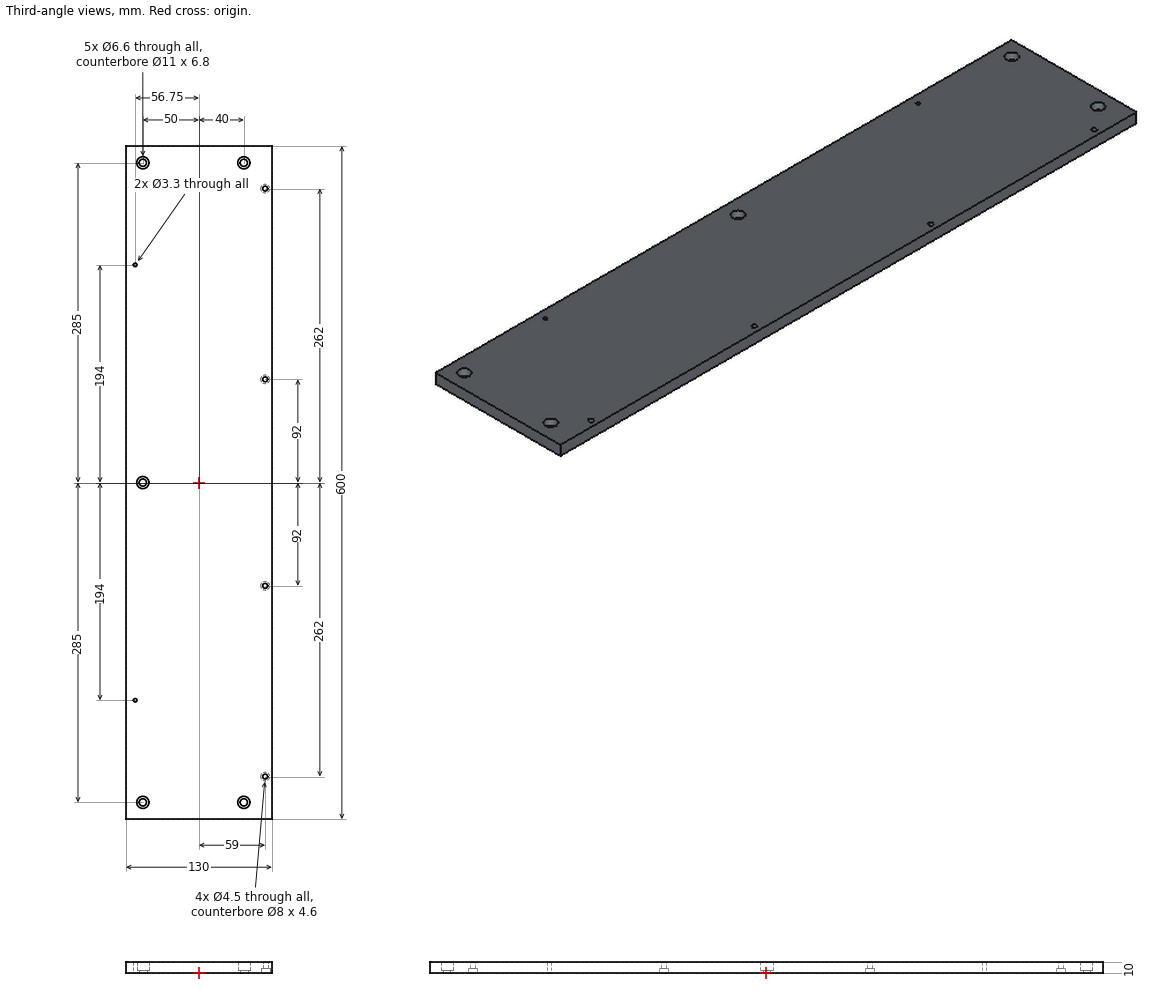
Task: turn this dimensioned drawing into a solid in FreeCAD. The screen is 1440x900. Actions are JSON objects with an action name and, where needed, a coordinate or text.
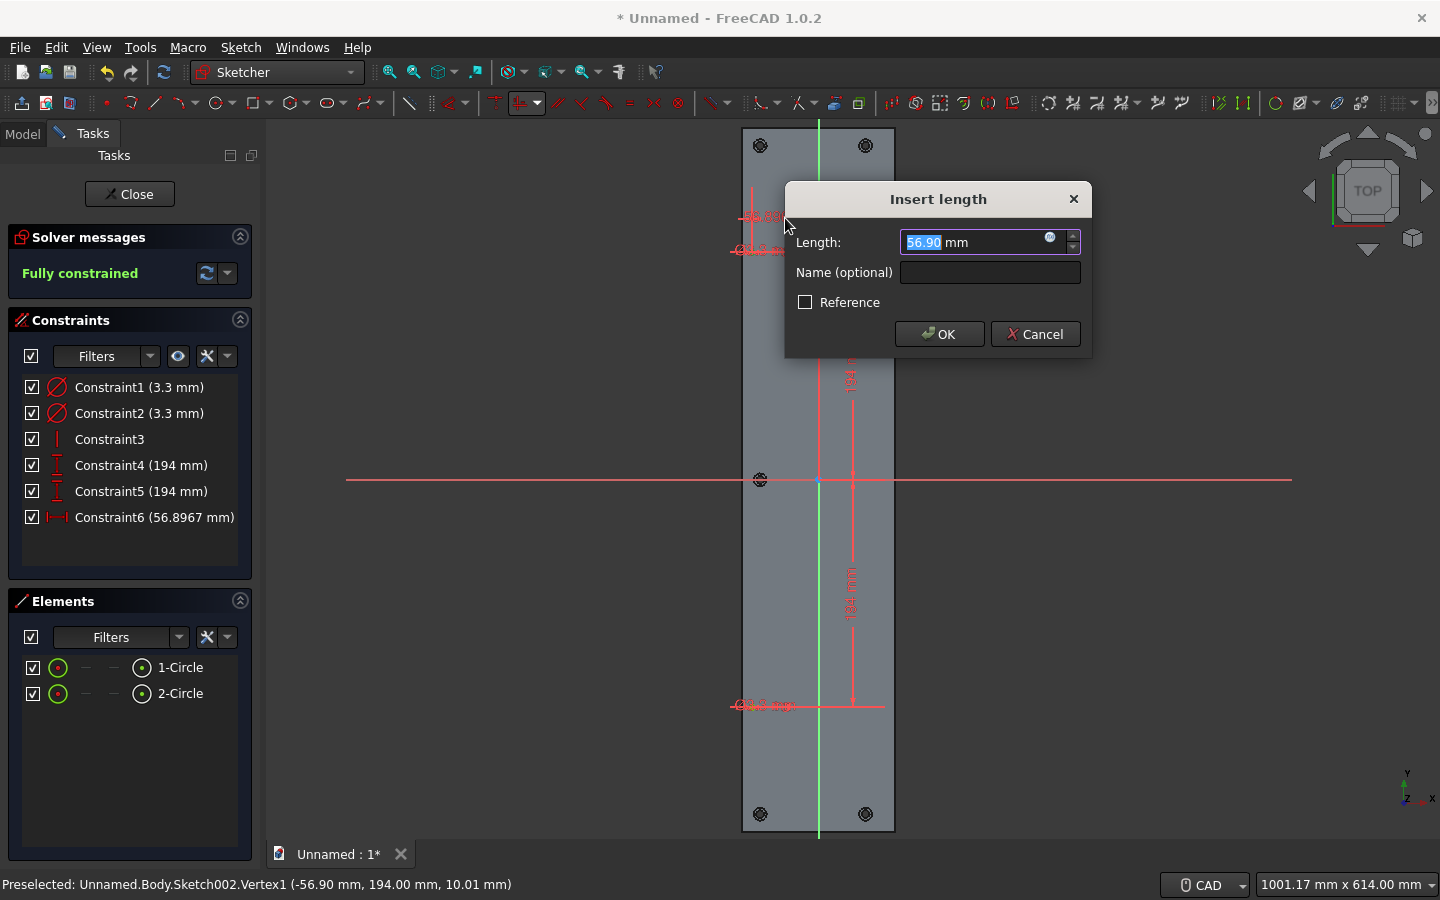
{"action": "type", "text": "56.75"}
{"action": "key", "text": "Return"}
{"action": "key", "text": "Escape"}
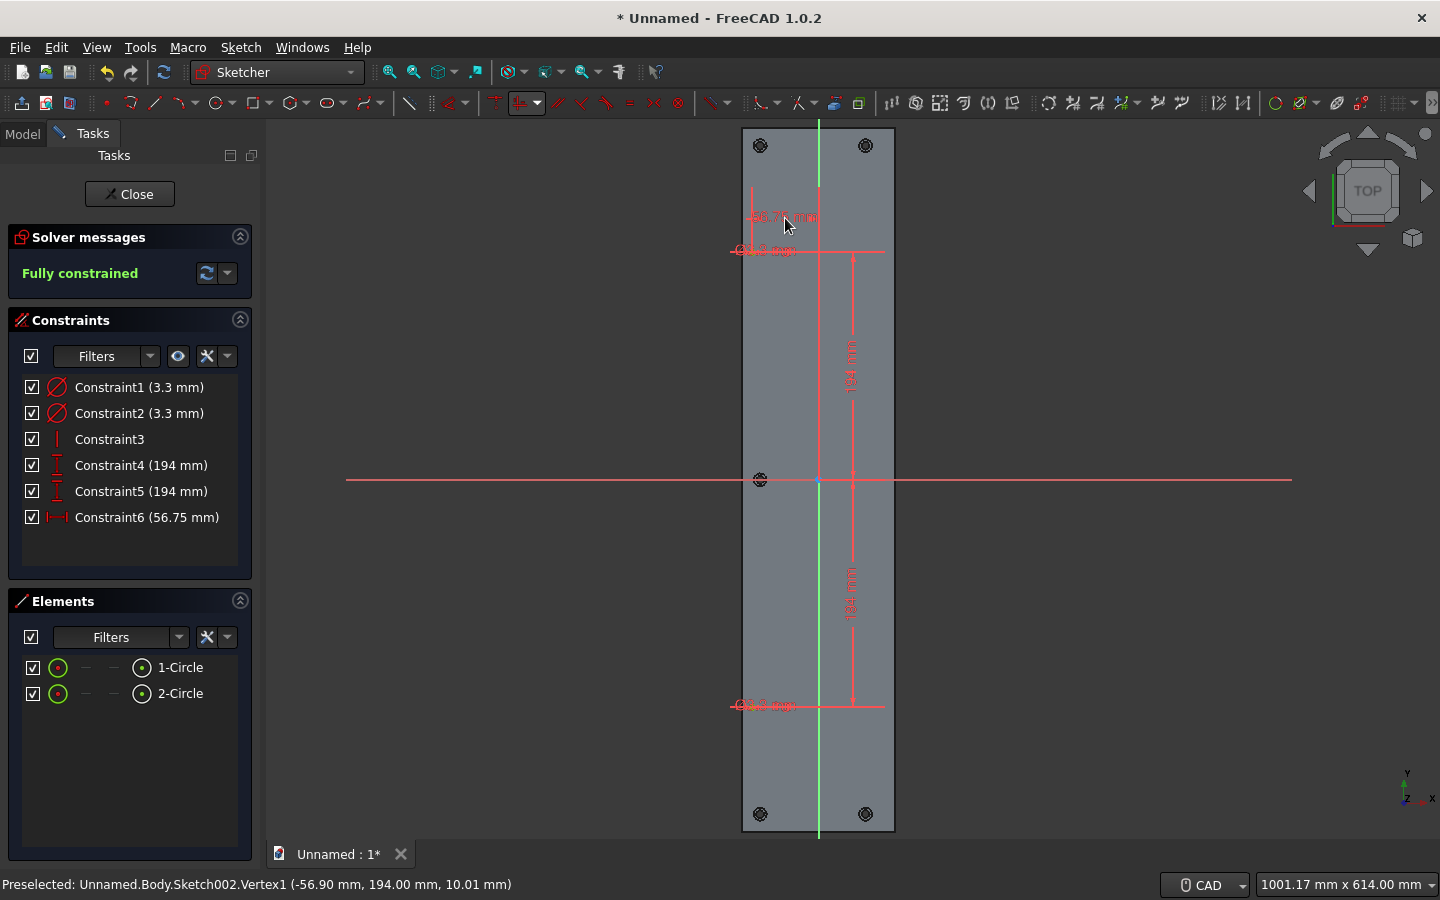
{"action": "left_click", "coordinate": [130, 194]}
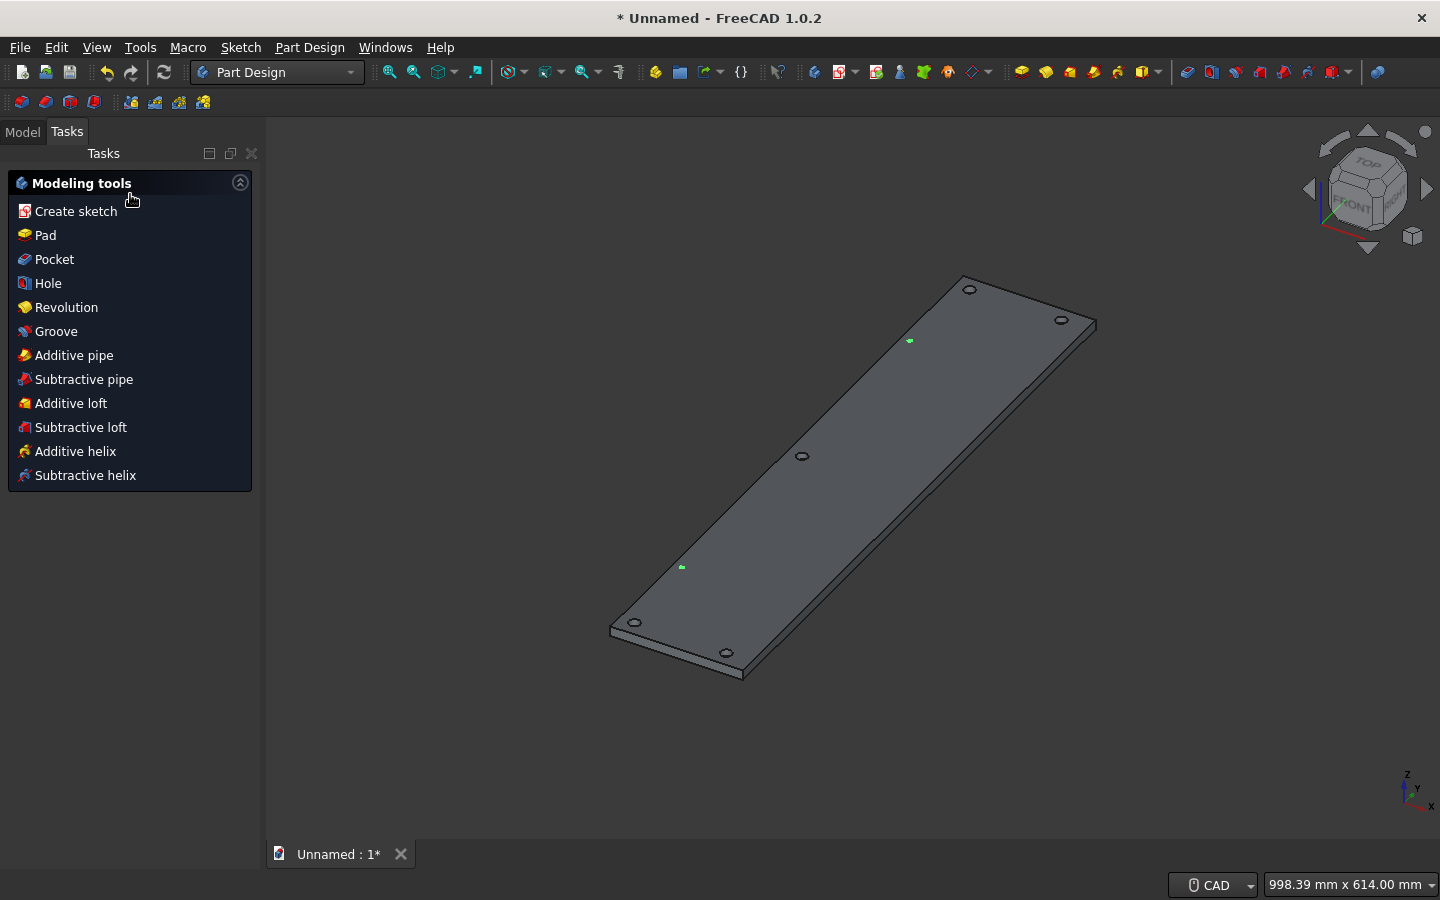
{"action": "left_click", "coordinate": [1212, 72]}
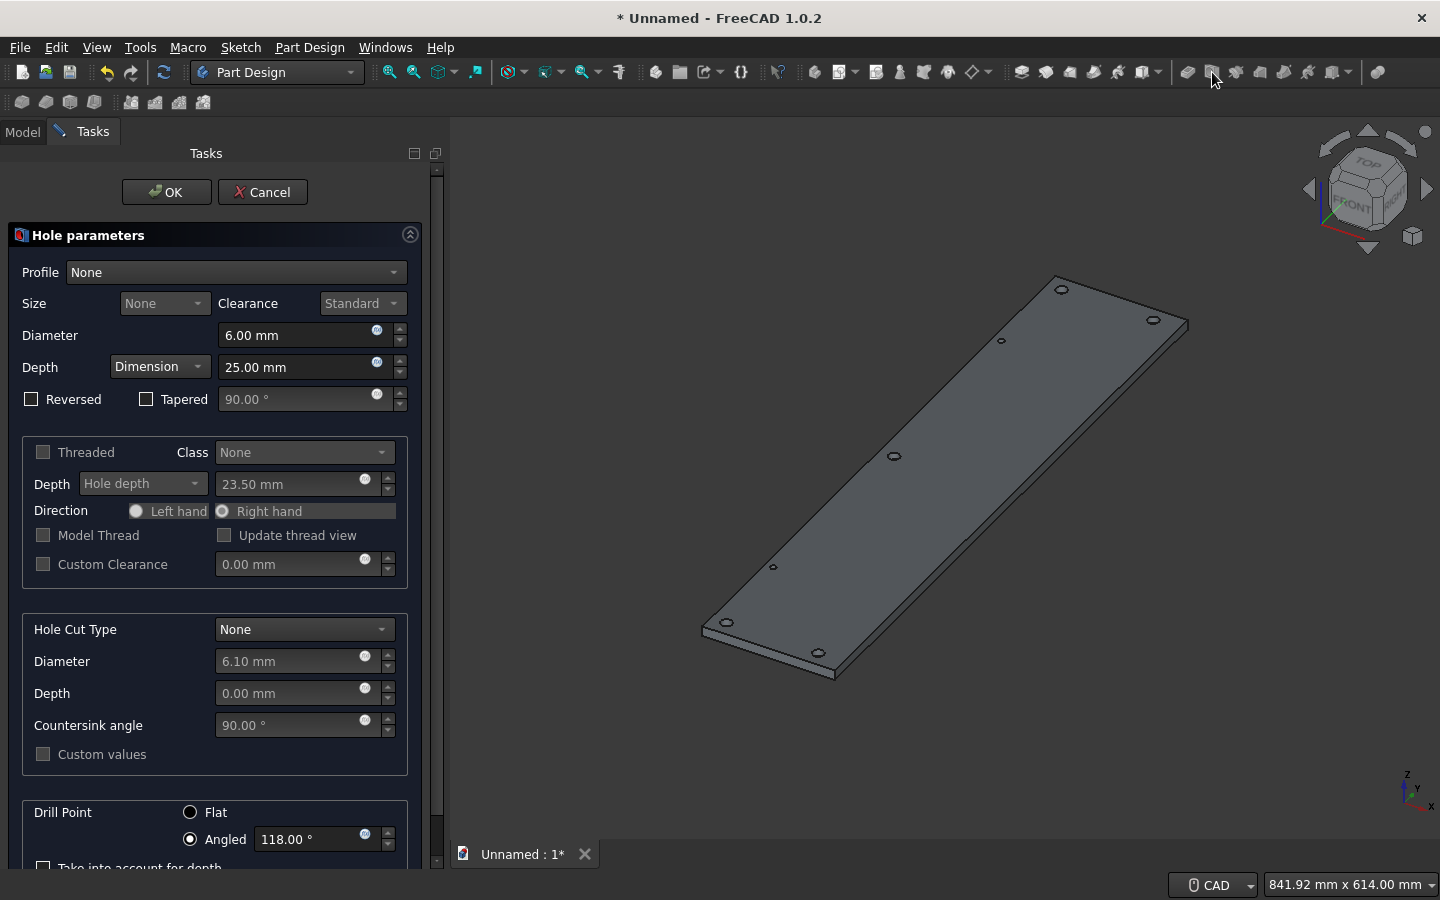
{"action": "triple_click", "coordinate": [305, 335]}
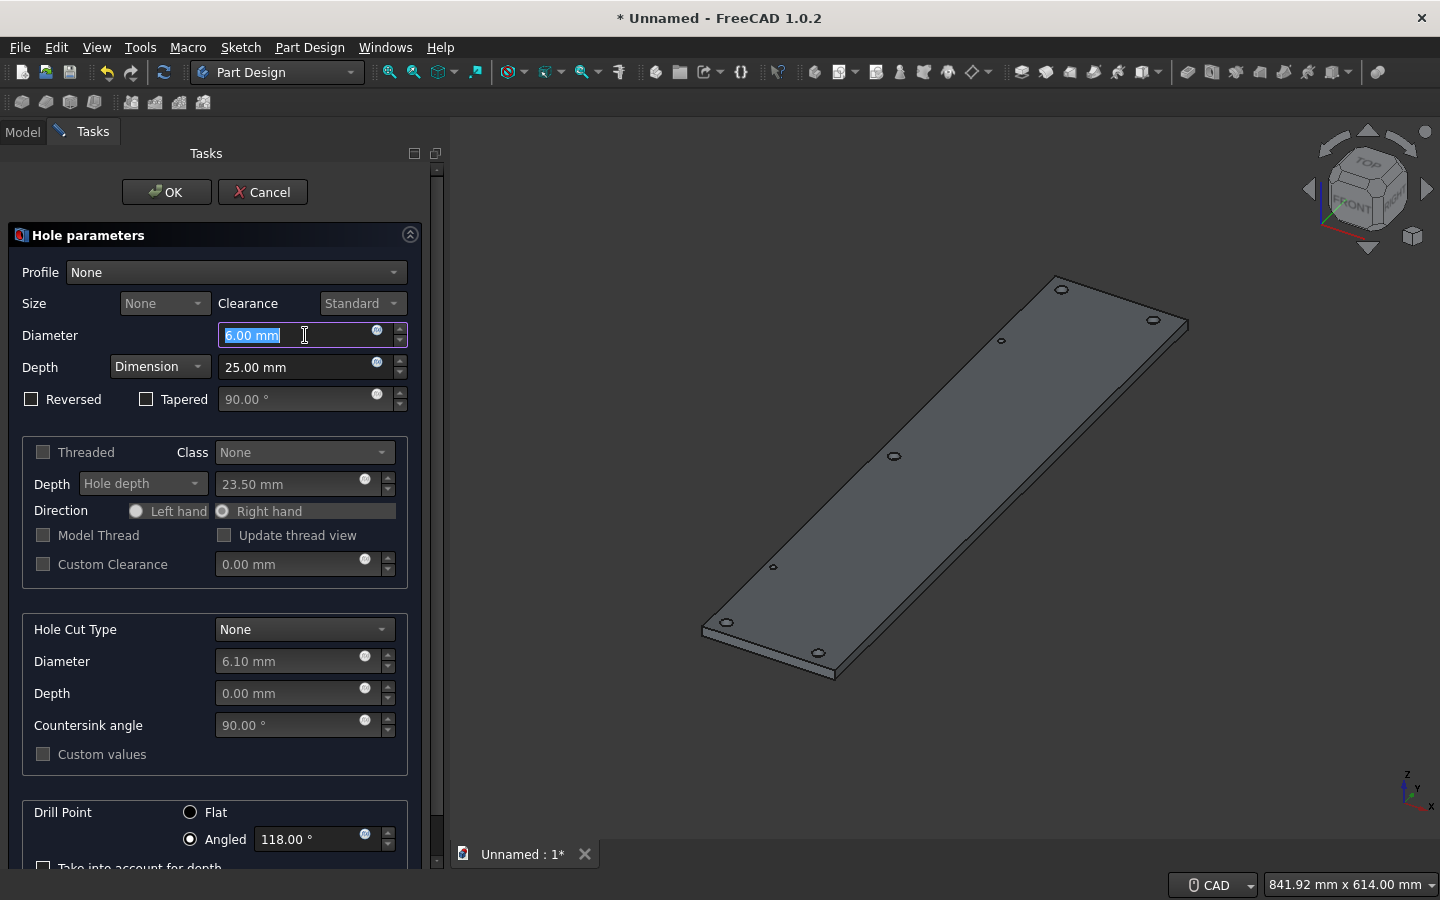
{"action": "type", "text": "3.3"}
{"action": "key", "text": "Tab"}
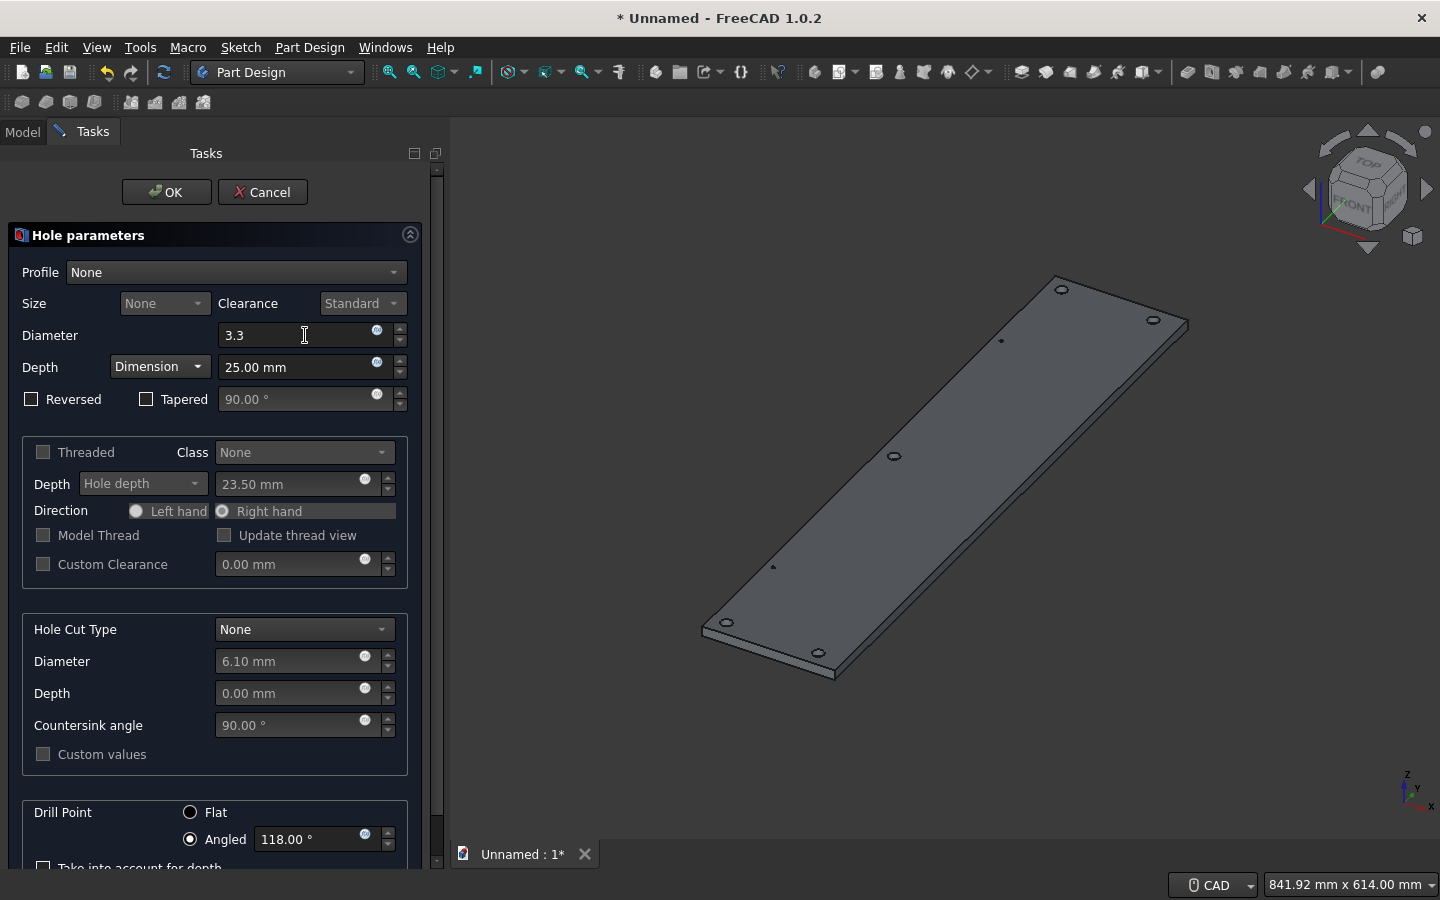
{"action": "left_click", "coordinate": [161, 366]}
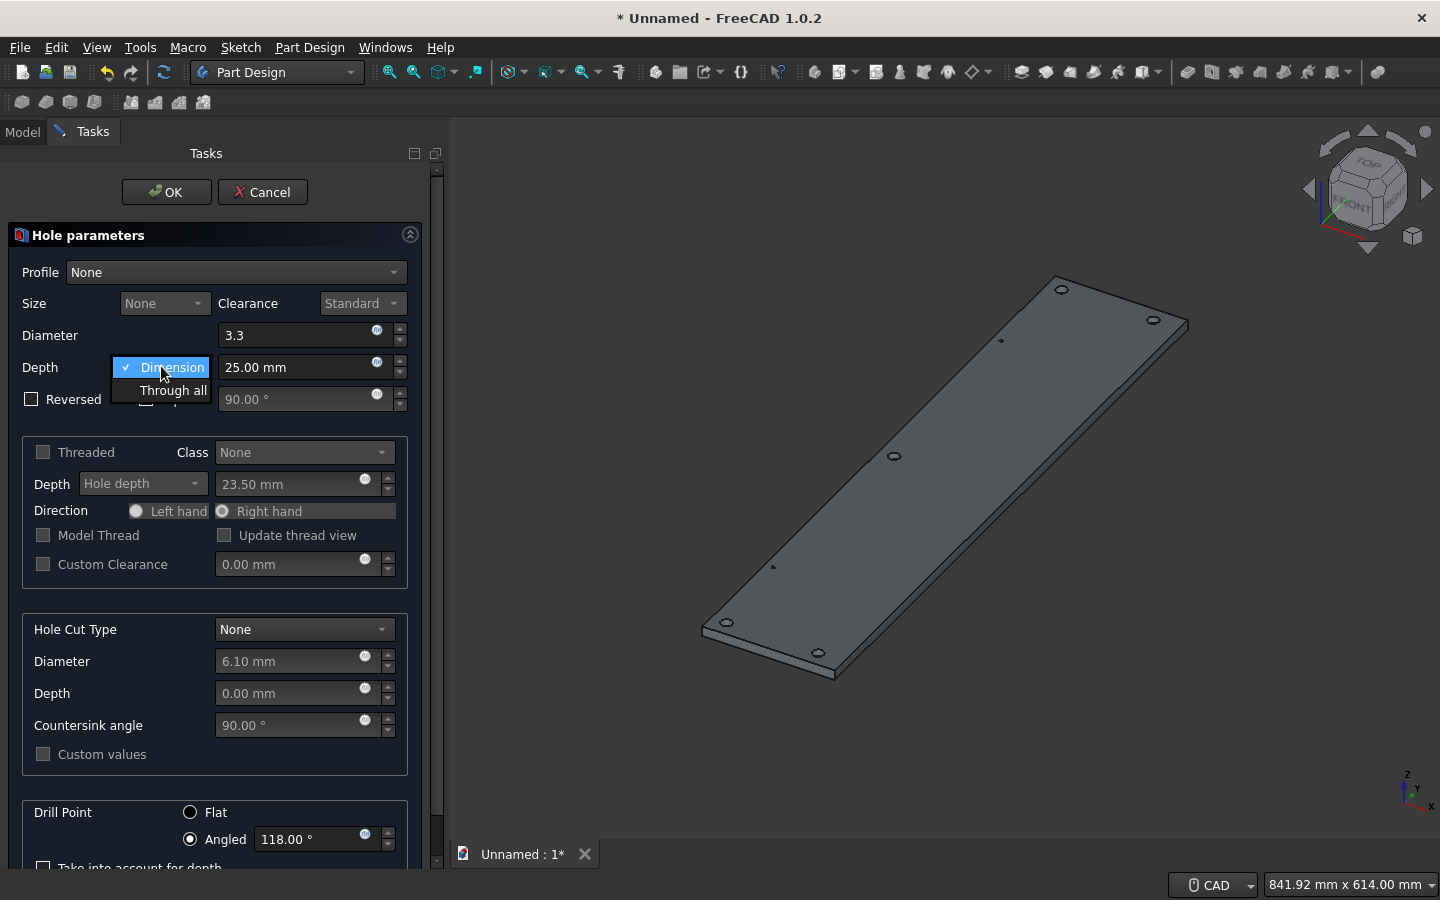
{"action": "left_click", "coordinate": [160, 390]}